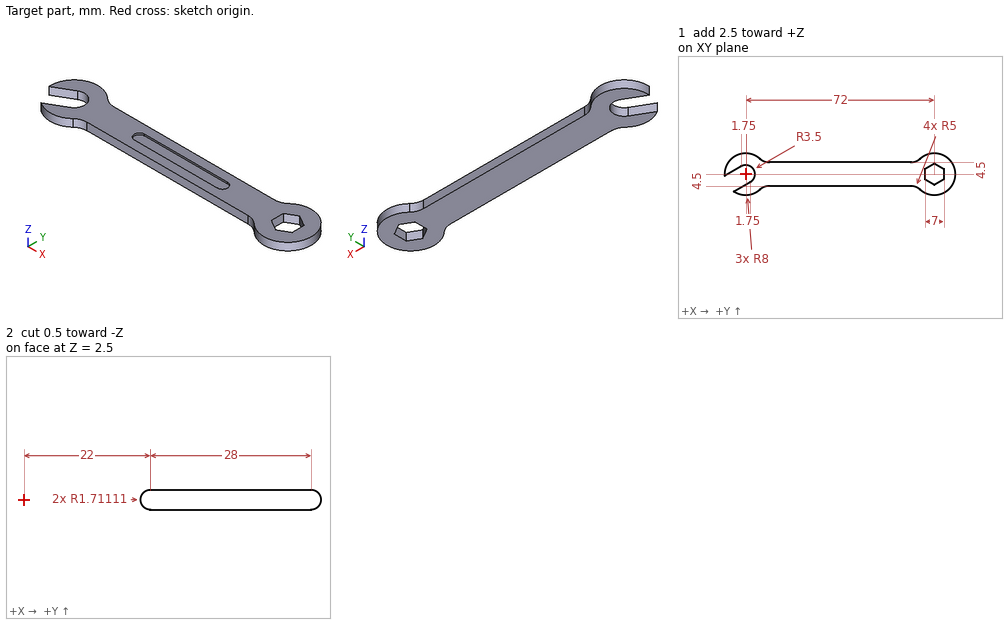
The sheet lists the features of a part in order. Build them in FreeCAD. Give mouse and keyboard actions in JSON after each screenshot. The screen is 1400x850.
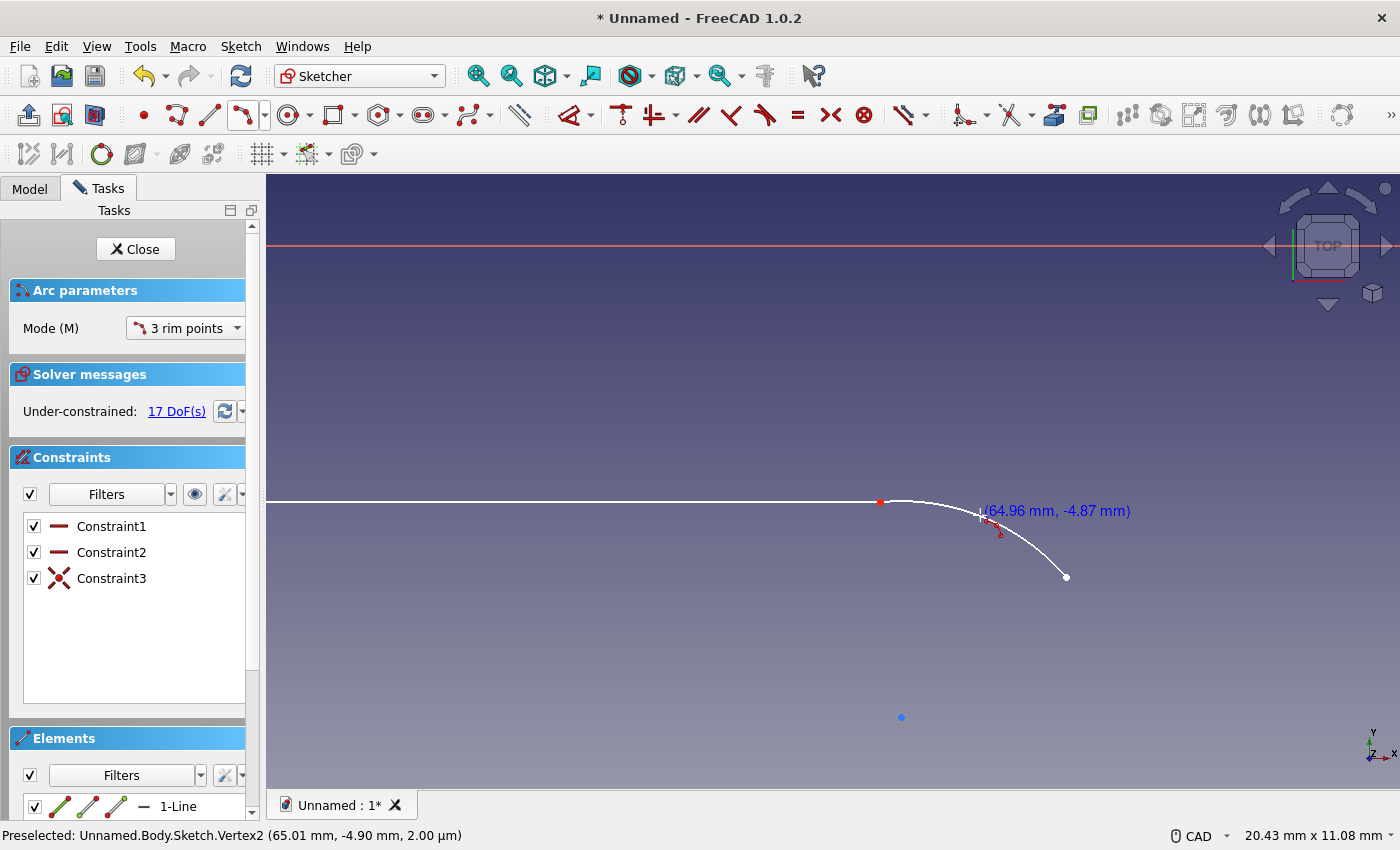
{"action": "scroll", "coordinate": [982, 515], "scroll_direction": "down", "scroll_amount": 10}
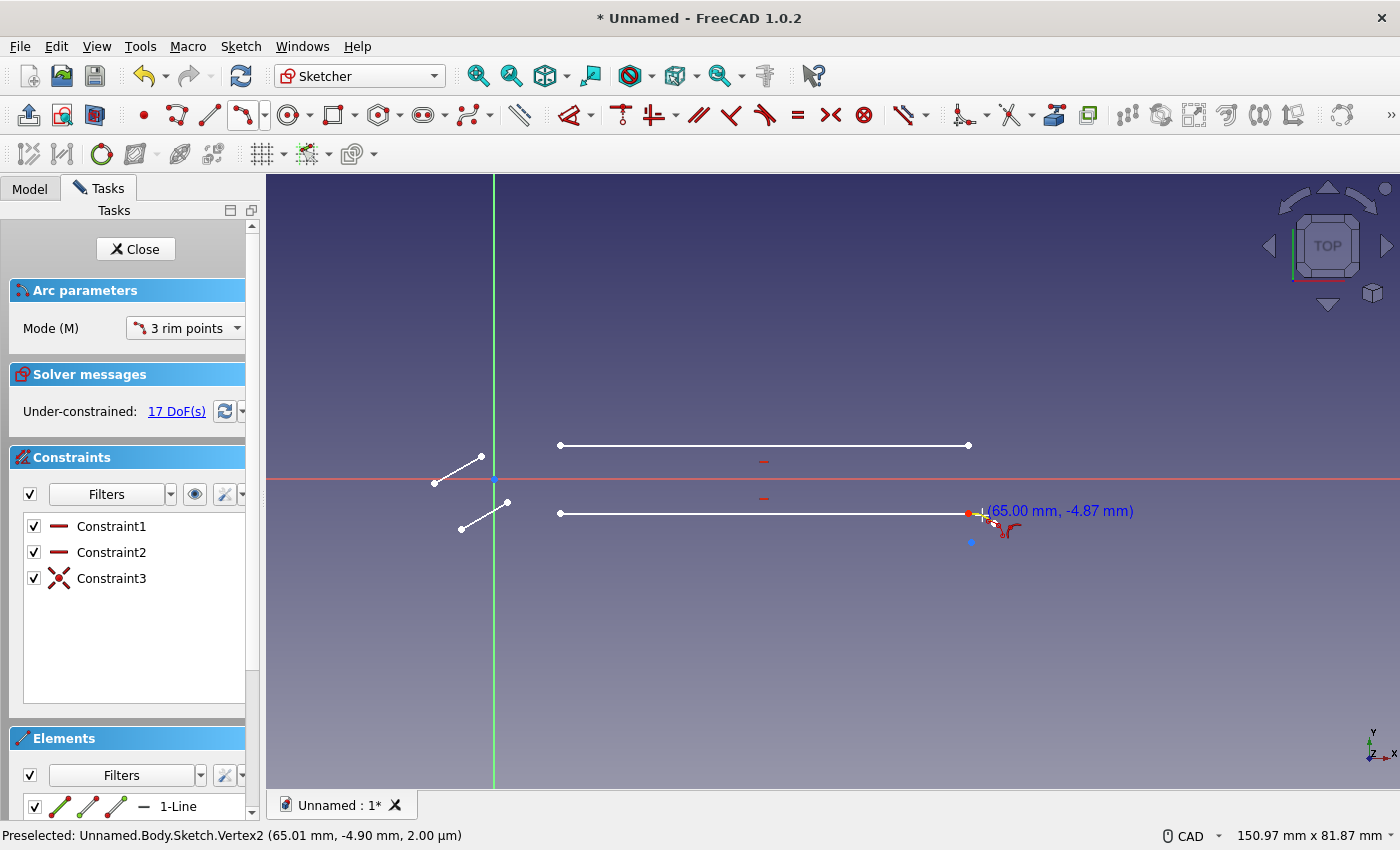
{"action": "left_click", "coordinate": [994, 524]}
{"action": "left_click", "coordinate": [994, 435]}
{"action": "left_click", "coordinate": [1089, 506]}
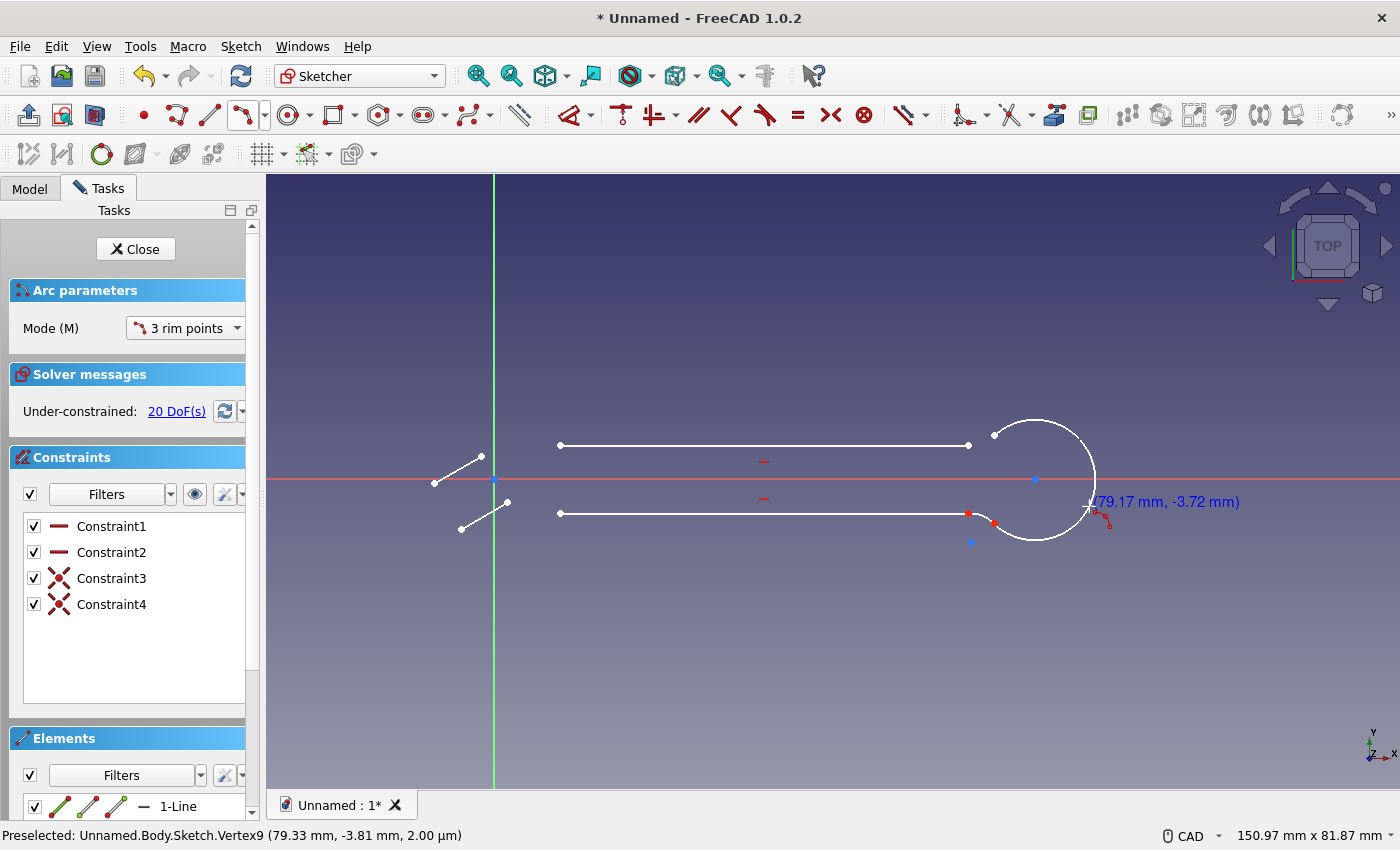
{"action": "left_click", "coordinate": [994, 436]}
{"action": "left_click", "coordinate": [969, 446]}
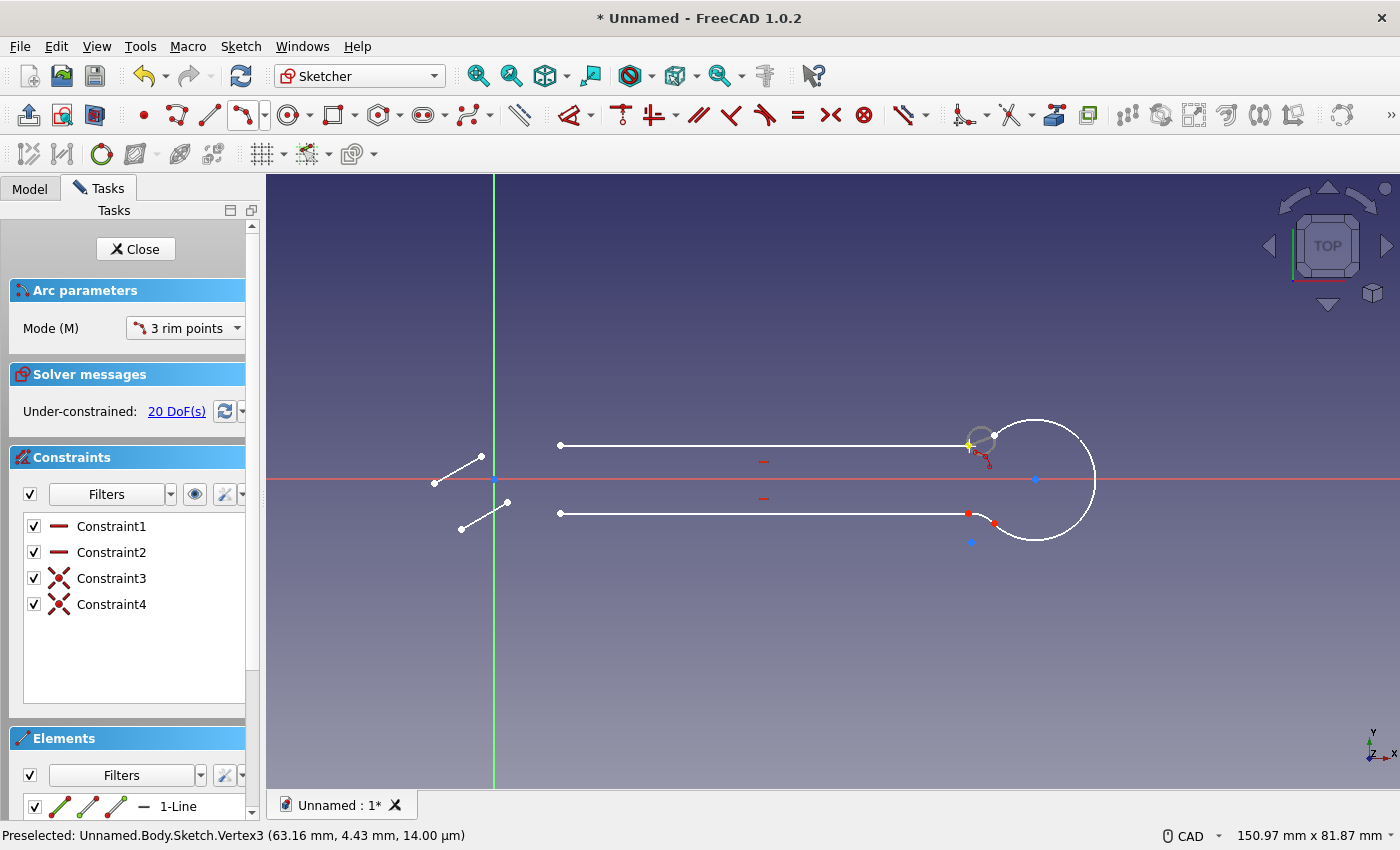
{"action": "scroll", "coordinate": [982, 443], "scroll_direction": "up", "scroll_amount": 10}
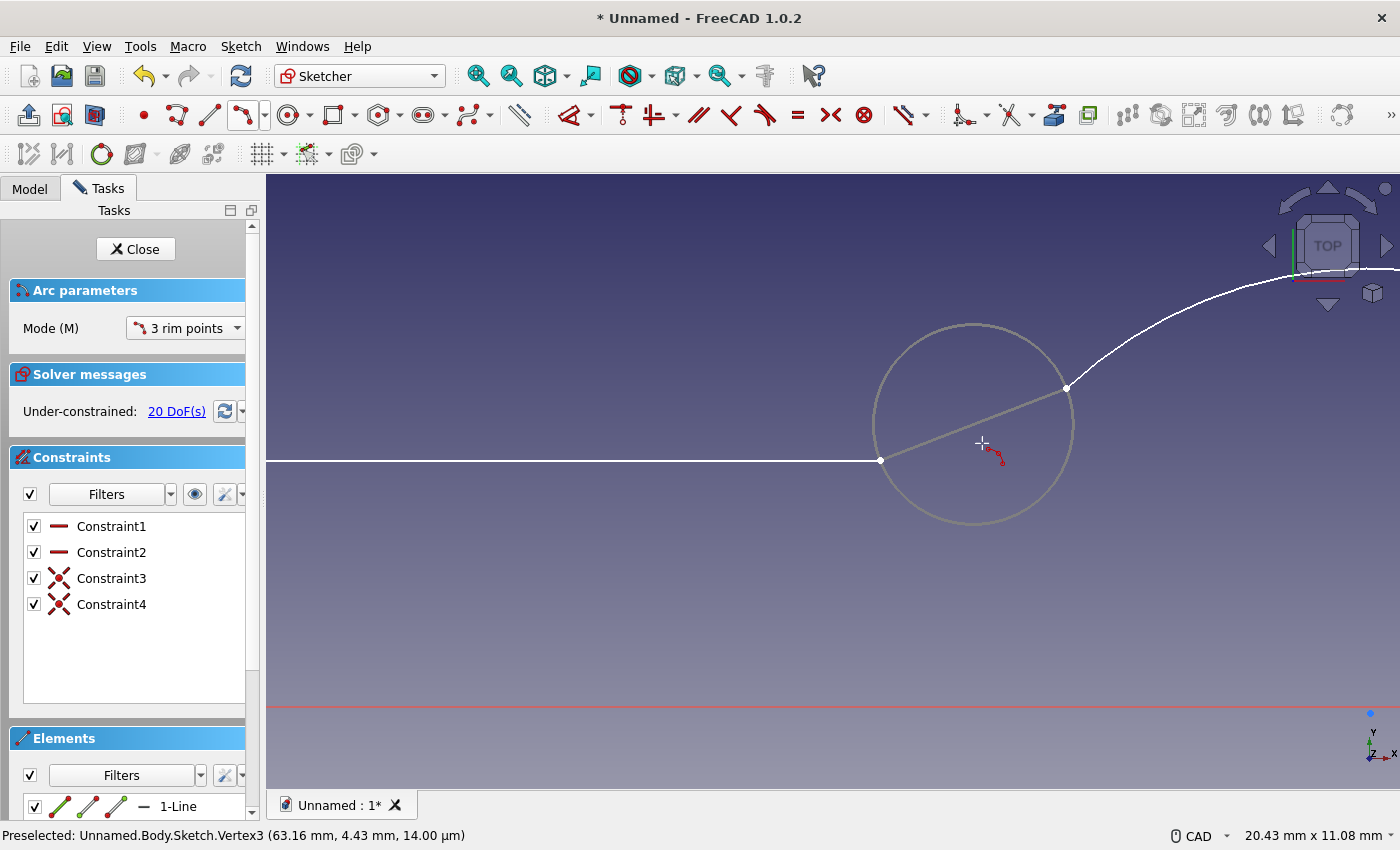
{"action": "left_click", "coordinate": [980, 437]}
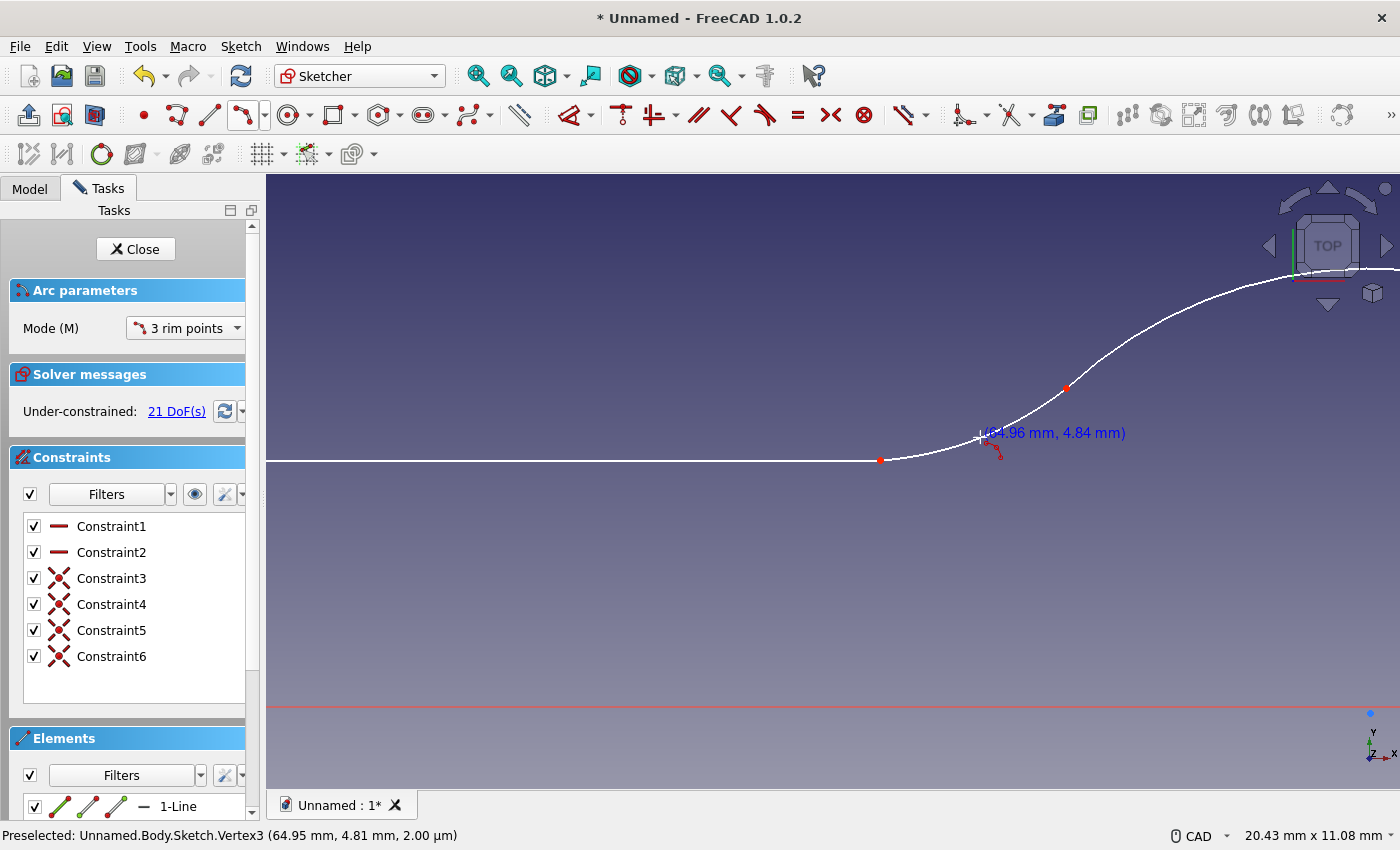
{"action": "scroll", "coordinate": [982, 443], "scroll_direction": "down", "scroll_amount": 10}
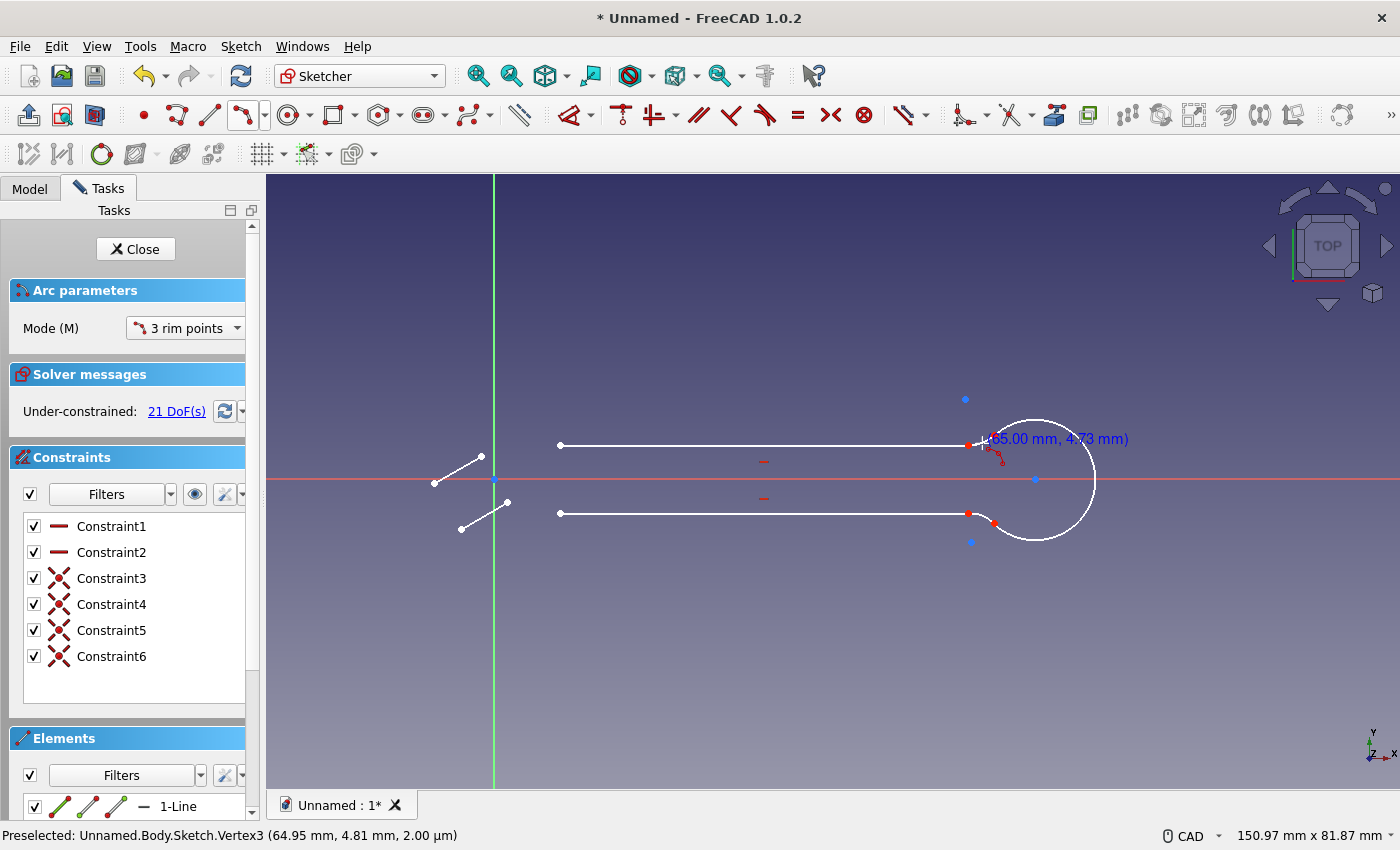
{"action": "left_click", "coordinate": [561, 446]}
{"action": "left_click", "coordinate": [535, 435]}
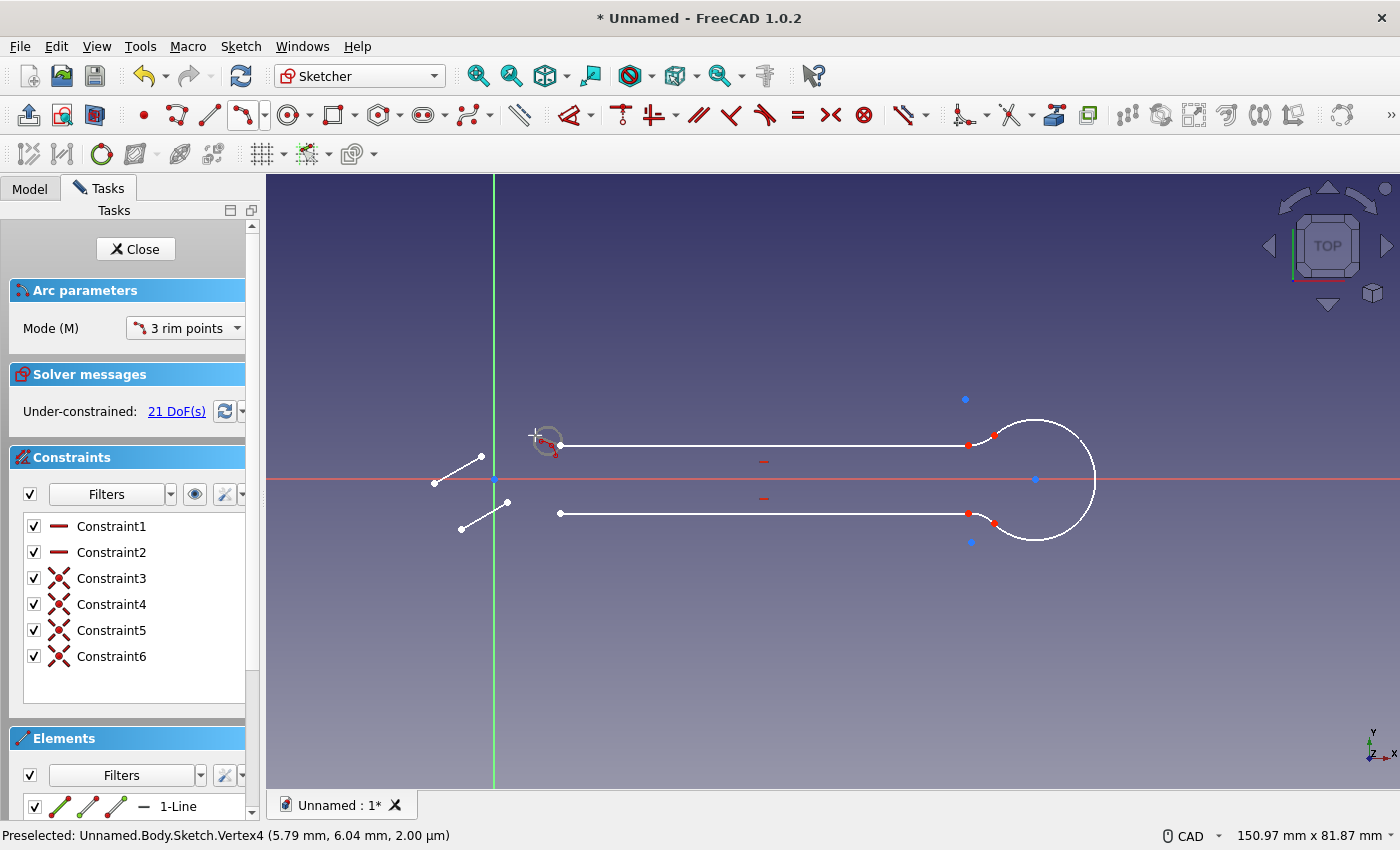
{"action": "scroll", "coordinate": [547, 443], "scroll_direction": "up", "scroll_amount": 10}